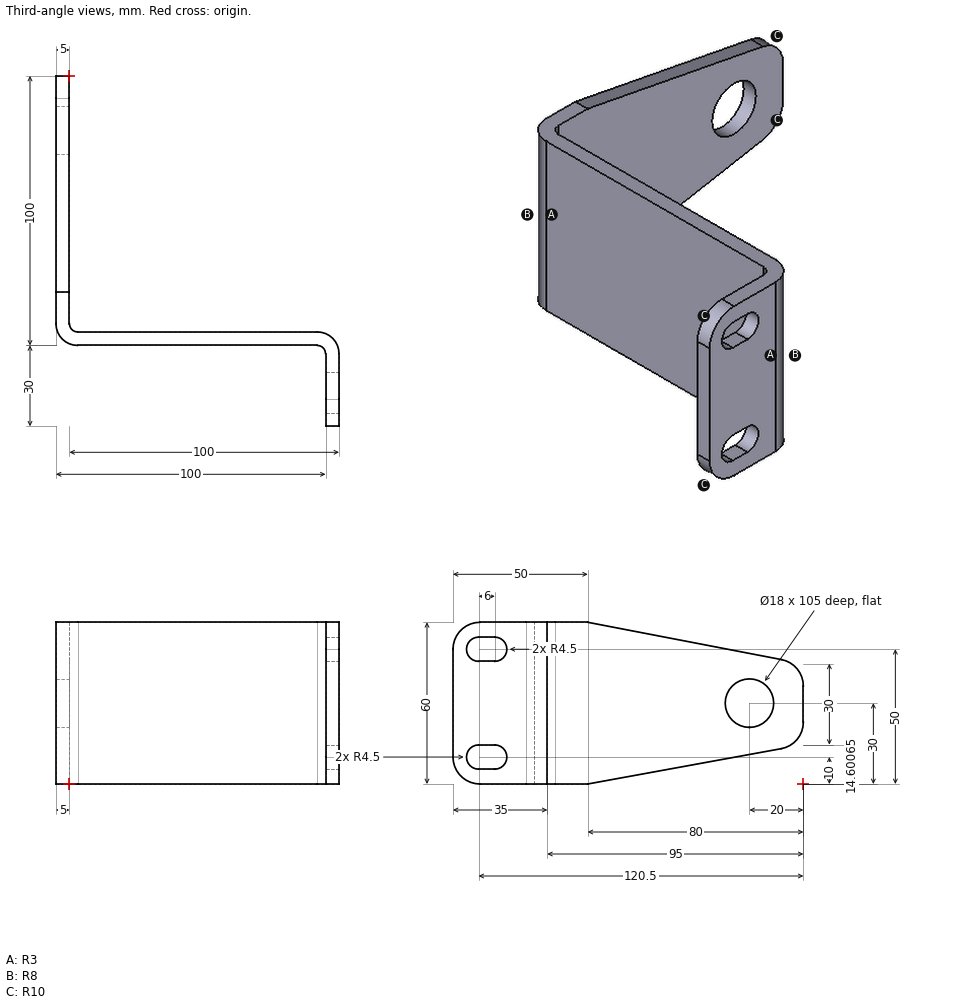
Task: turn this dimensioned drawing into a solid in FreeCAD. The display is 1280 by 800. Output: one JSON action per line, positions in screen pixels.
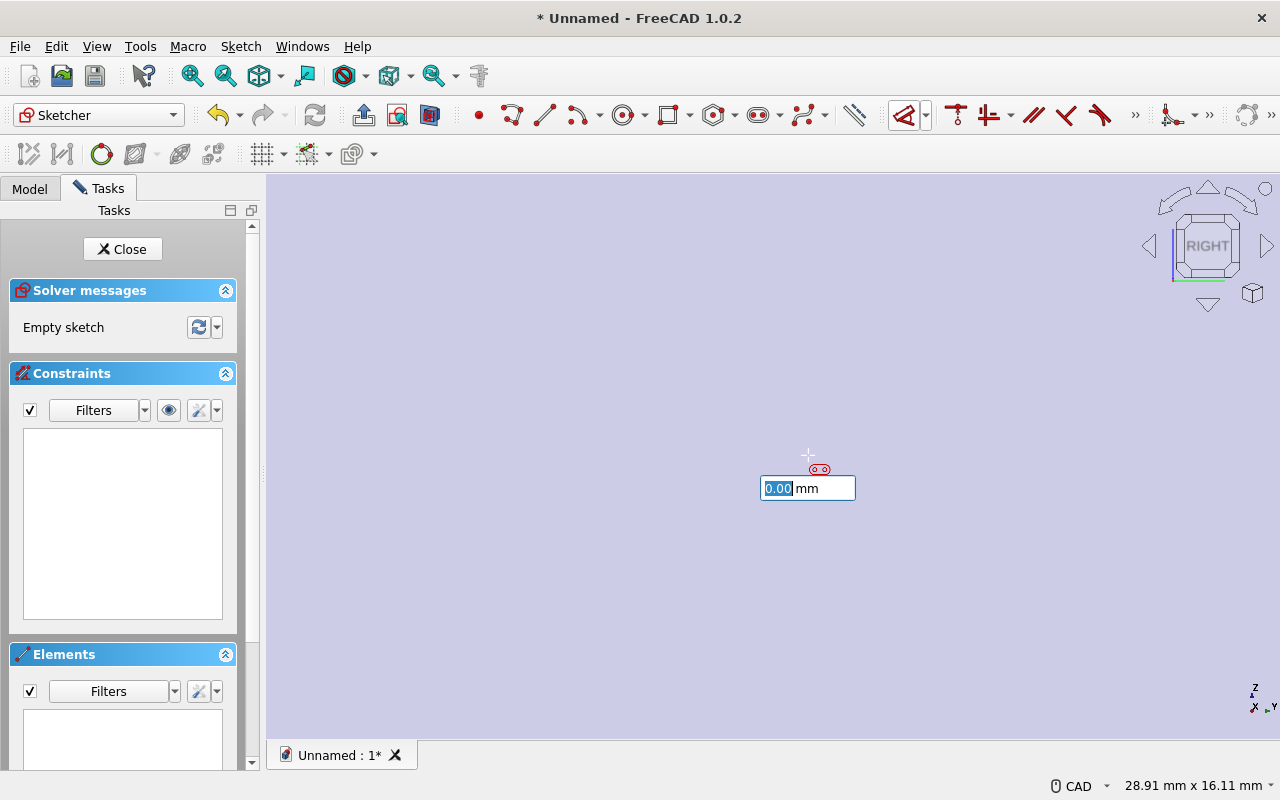
{"action": "left_click", "coordinate": [702, 297]}
{"action": "key", "text": "Escape"}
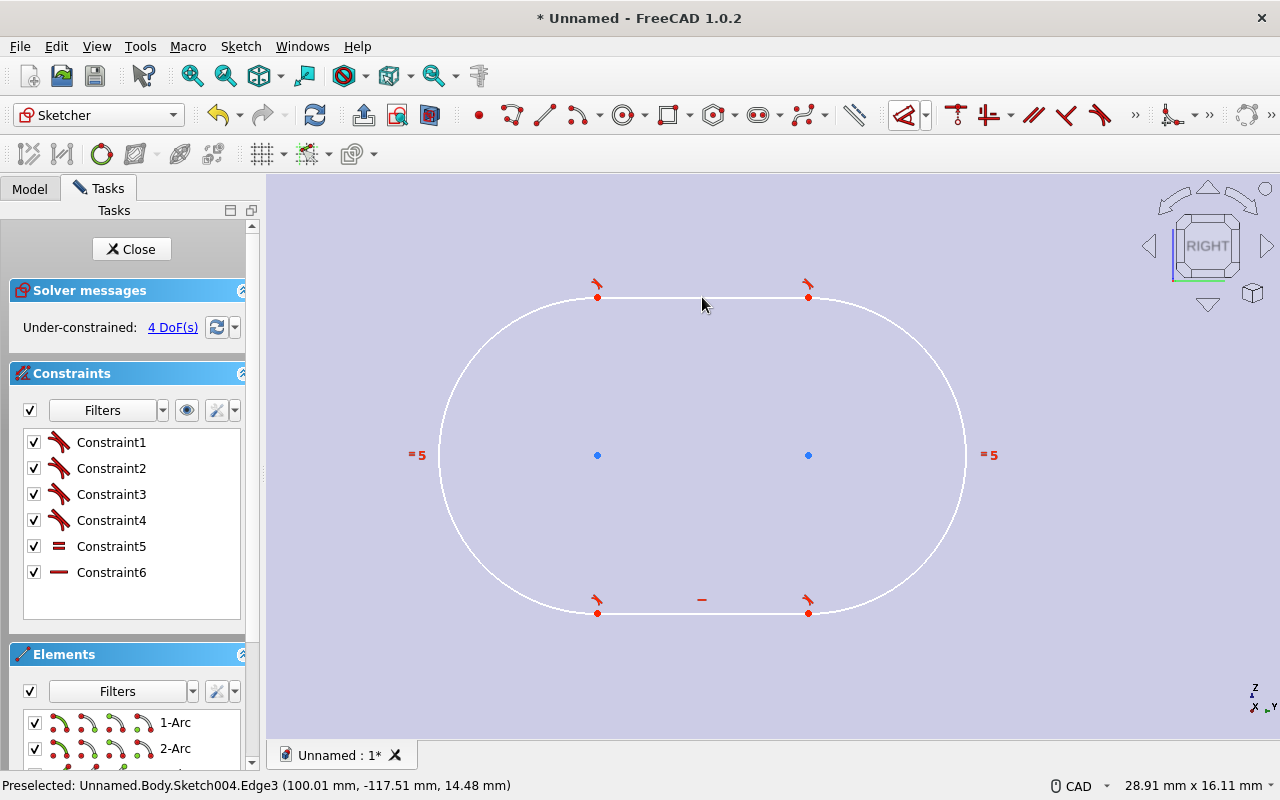
{"action": "left_click", "coordinate": [469, 363]}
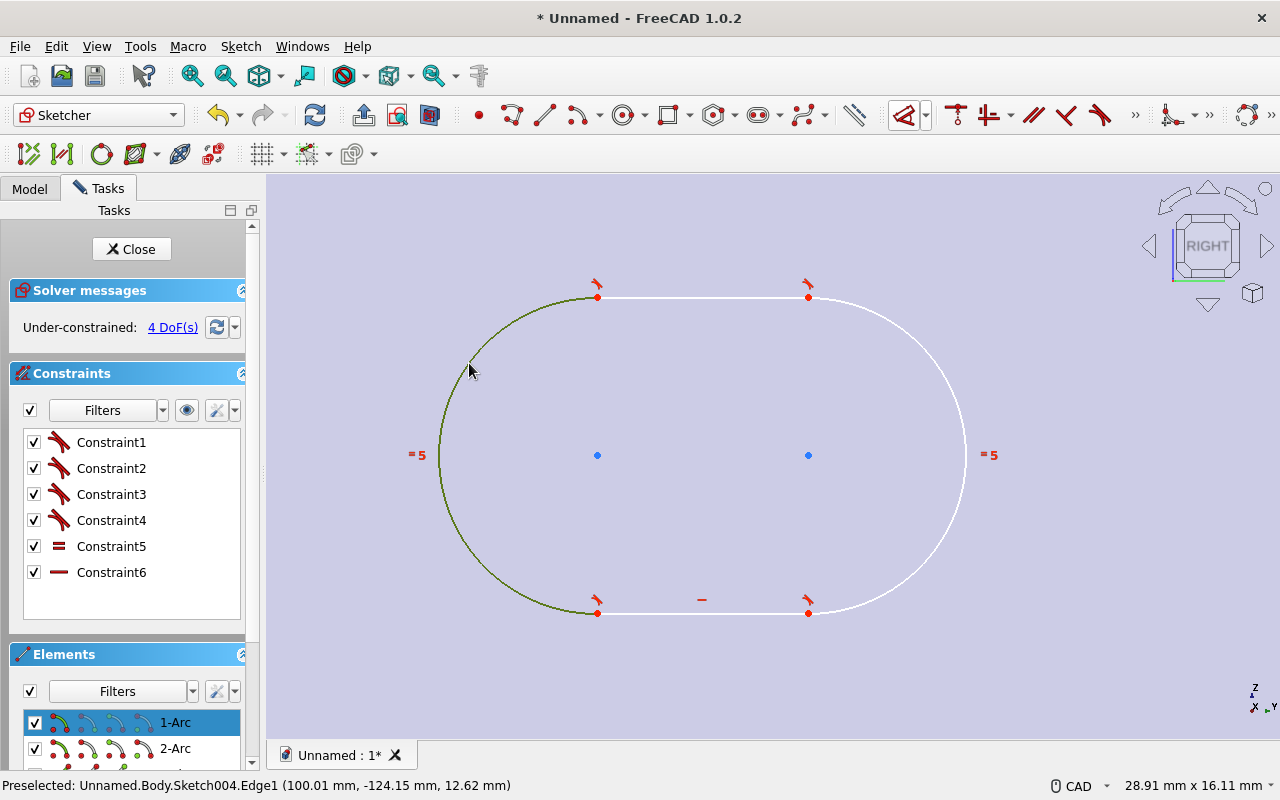
{"action": "left_click", "coordinate": [926, 116]}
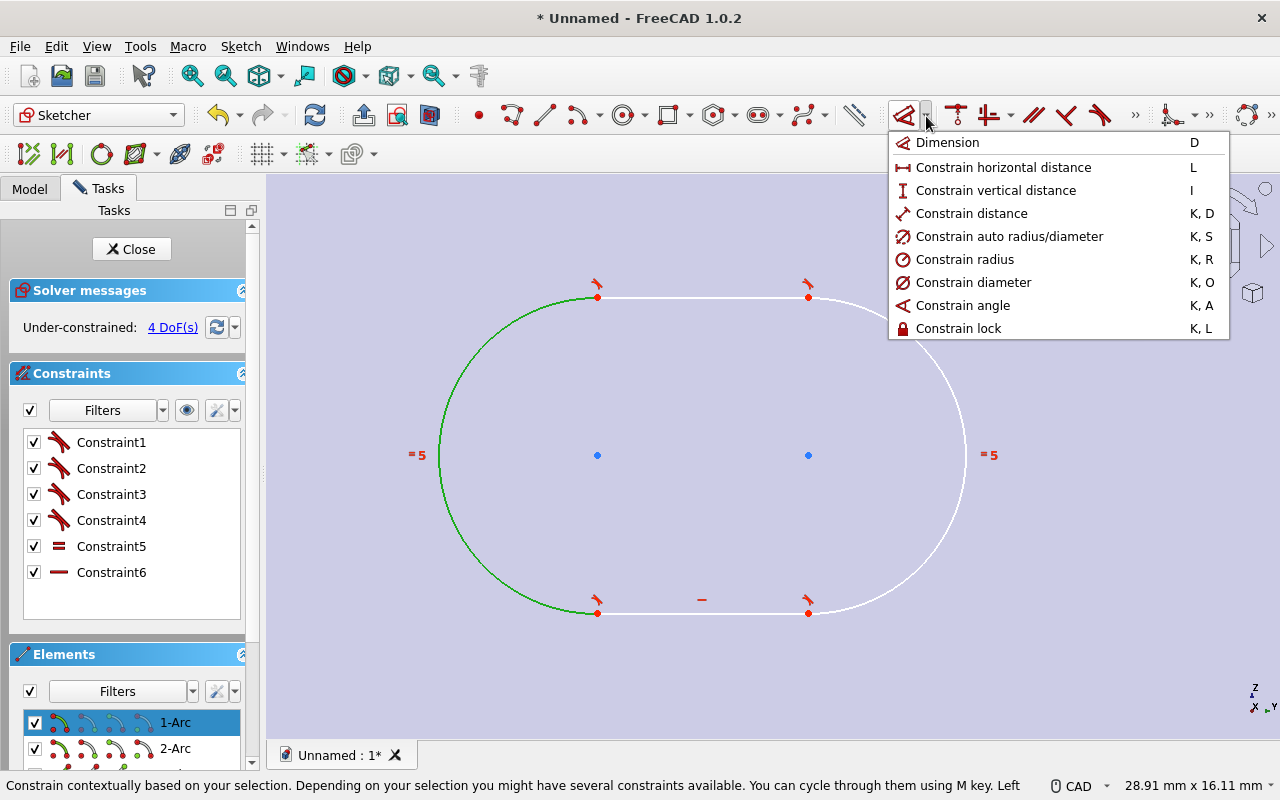
{"action": "left_click", "coordinate": [1059, 260]}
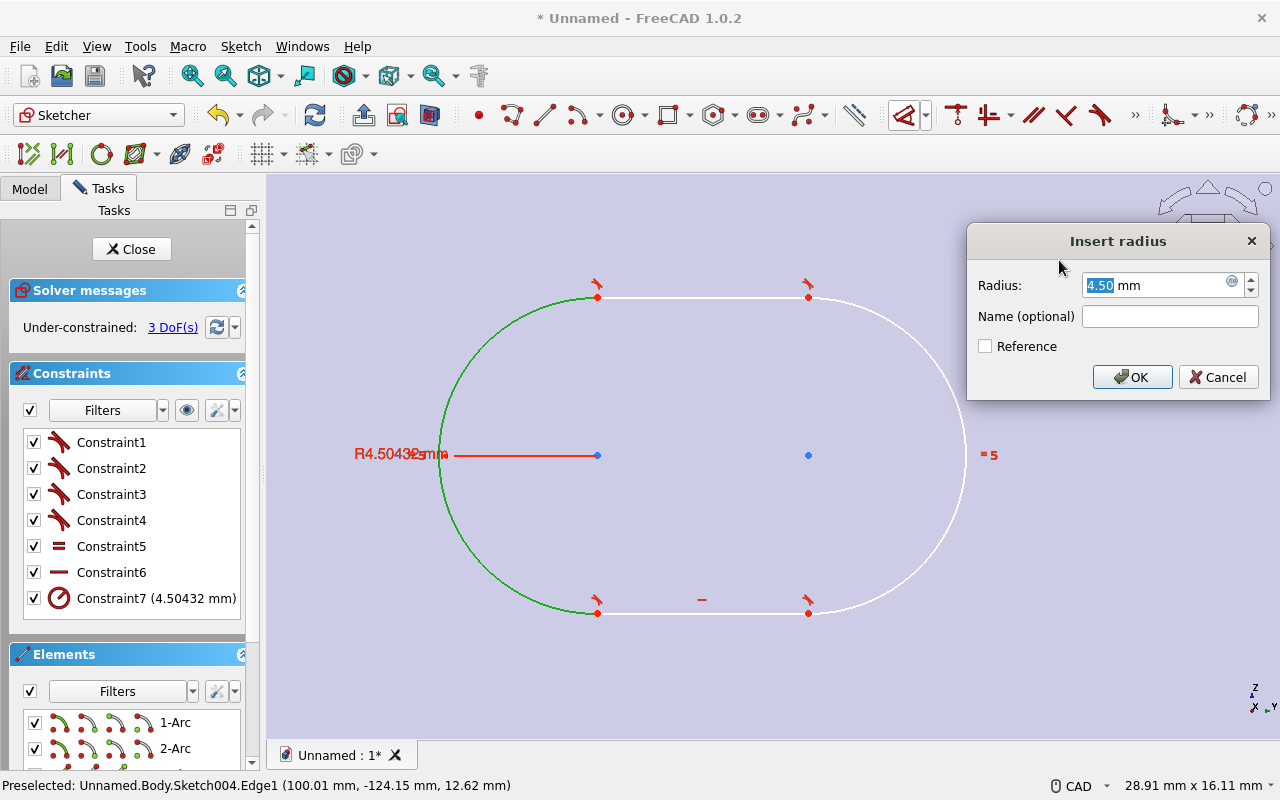
{"action": "type", "text": "4.5"}
{"action": "key", "text": "Return"}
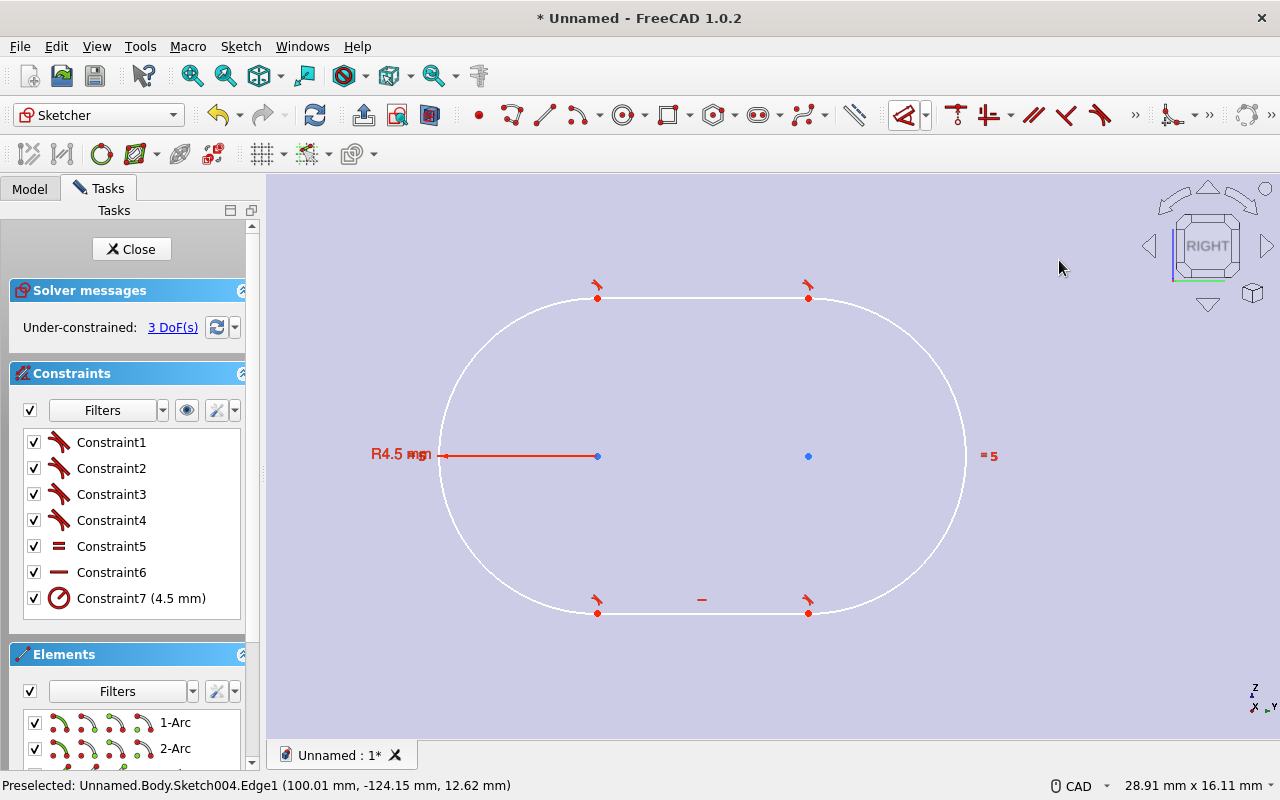
{"action": "left_click", "coordinate": [660, 298]}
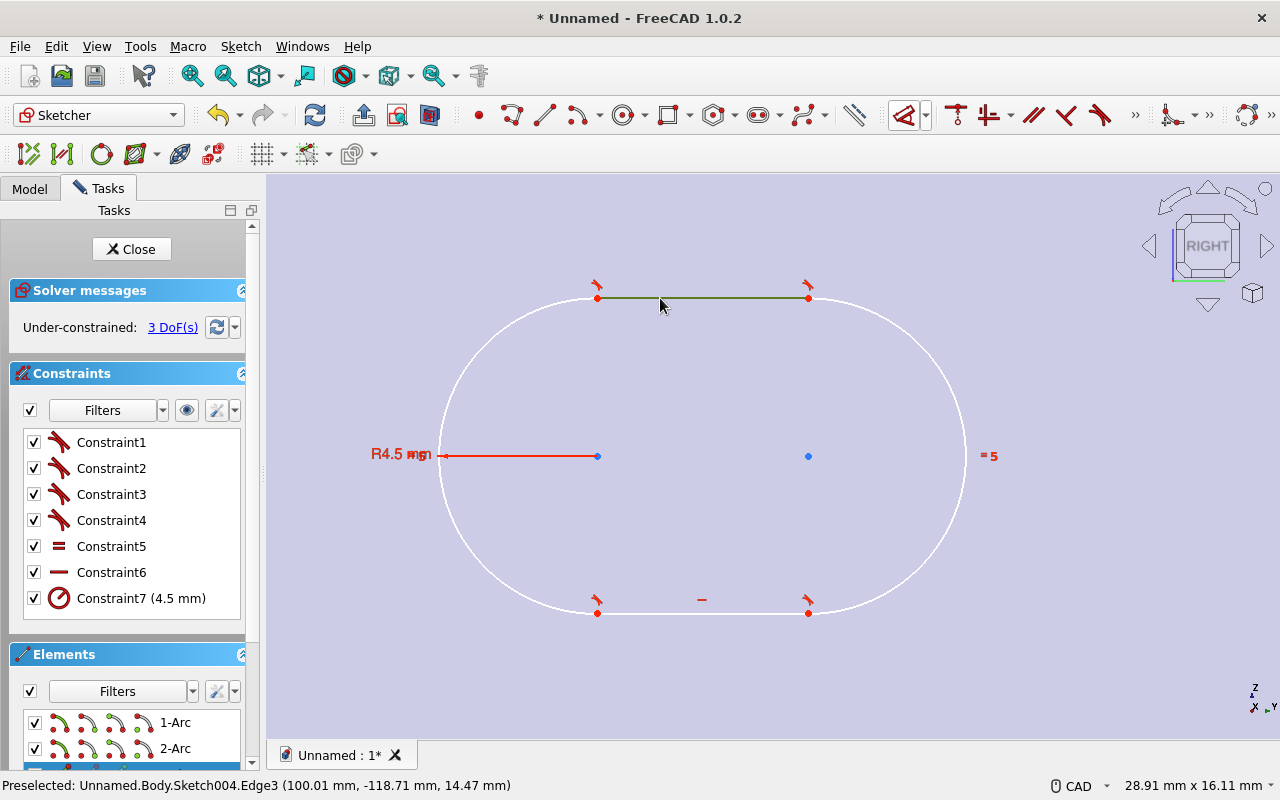
{"action": "key", "text": "l"}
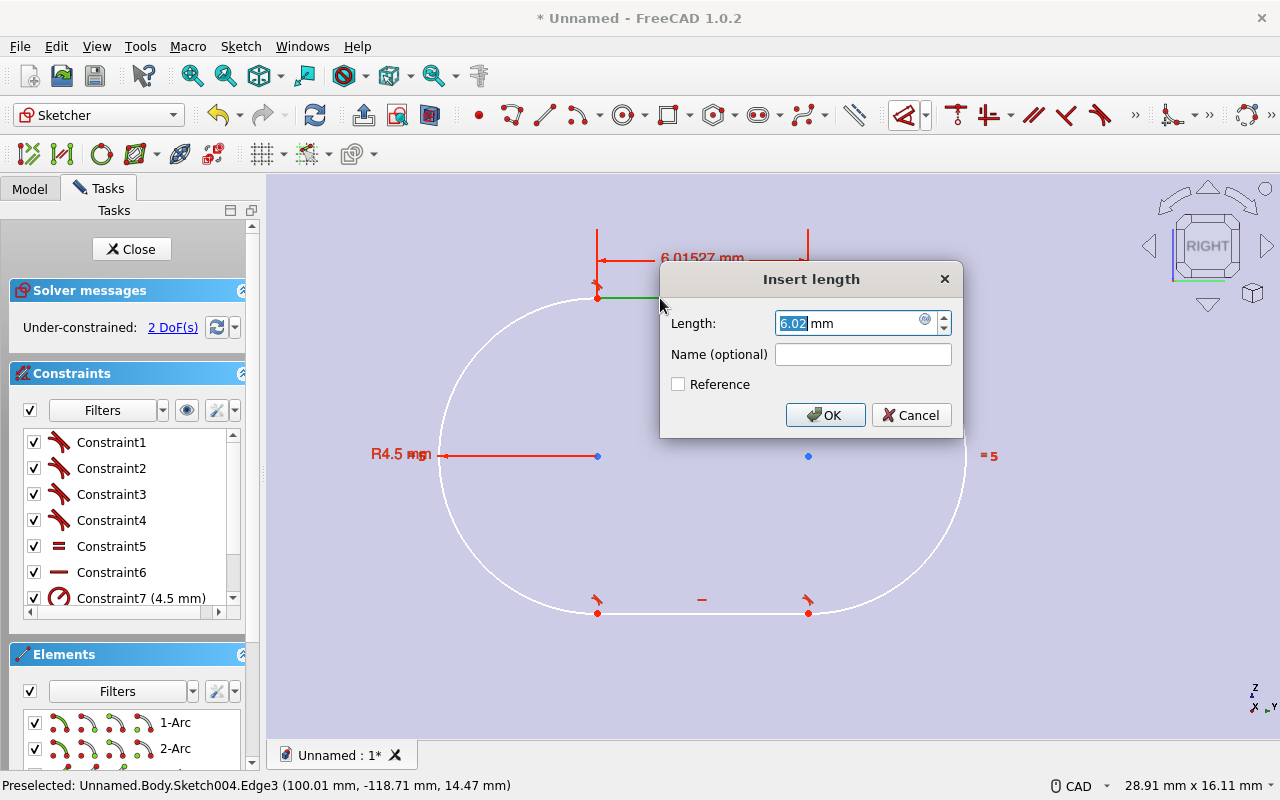
{"action": "type", "text": "6"}
{"action": "key", "text": "Return"}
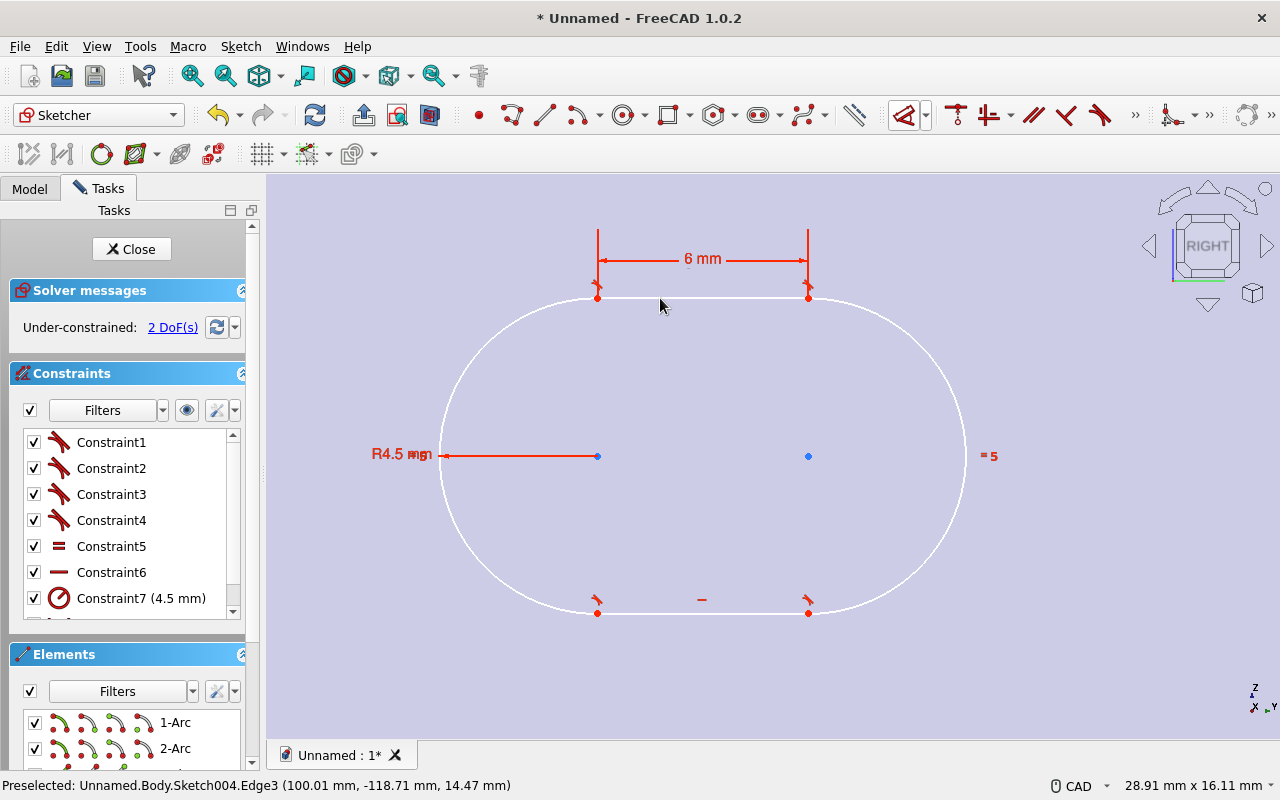
{"action": "left_click", "coordinate": [598, 456]}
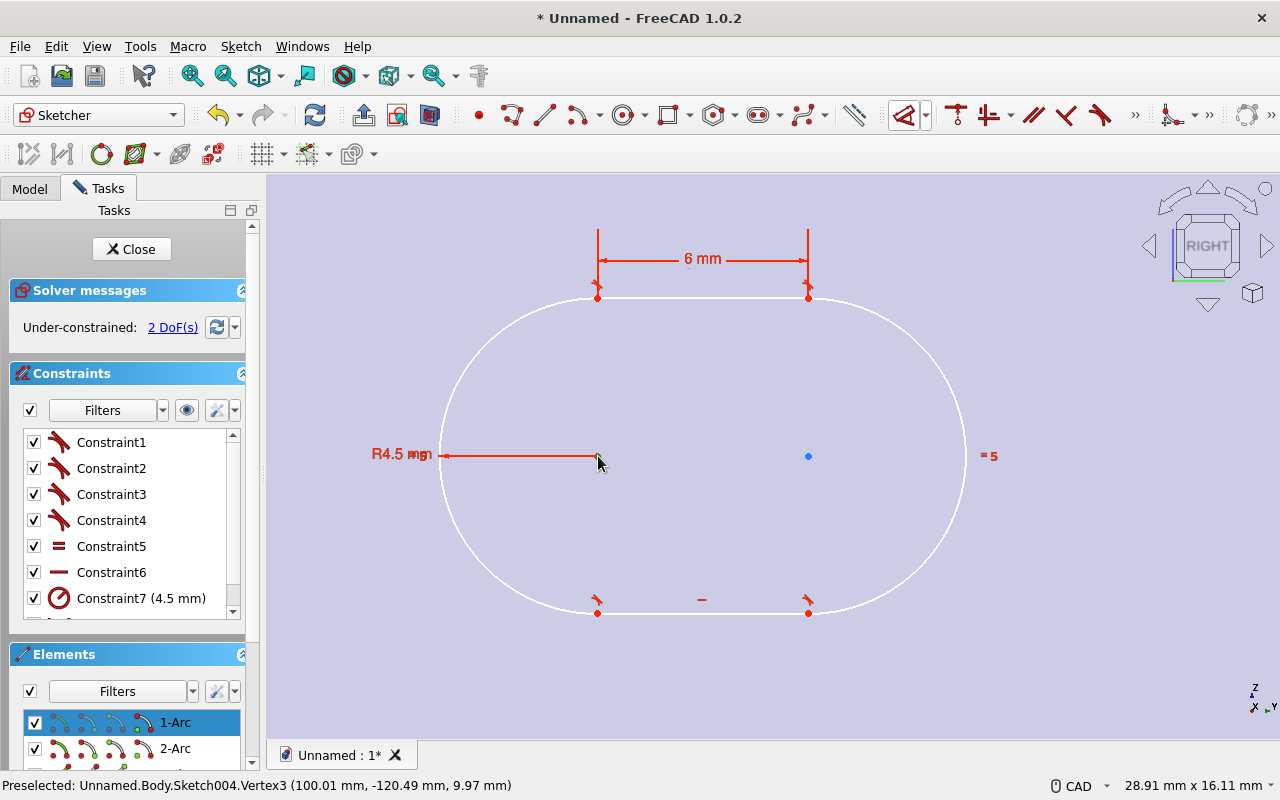
{"action": "left_click", "coordinate": [926, 116]}